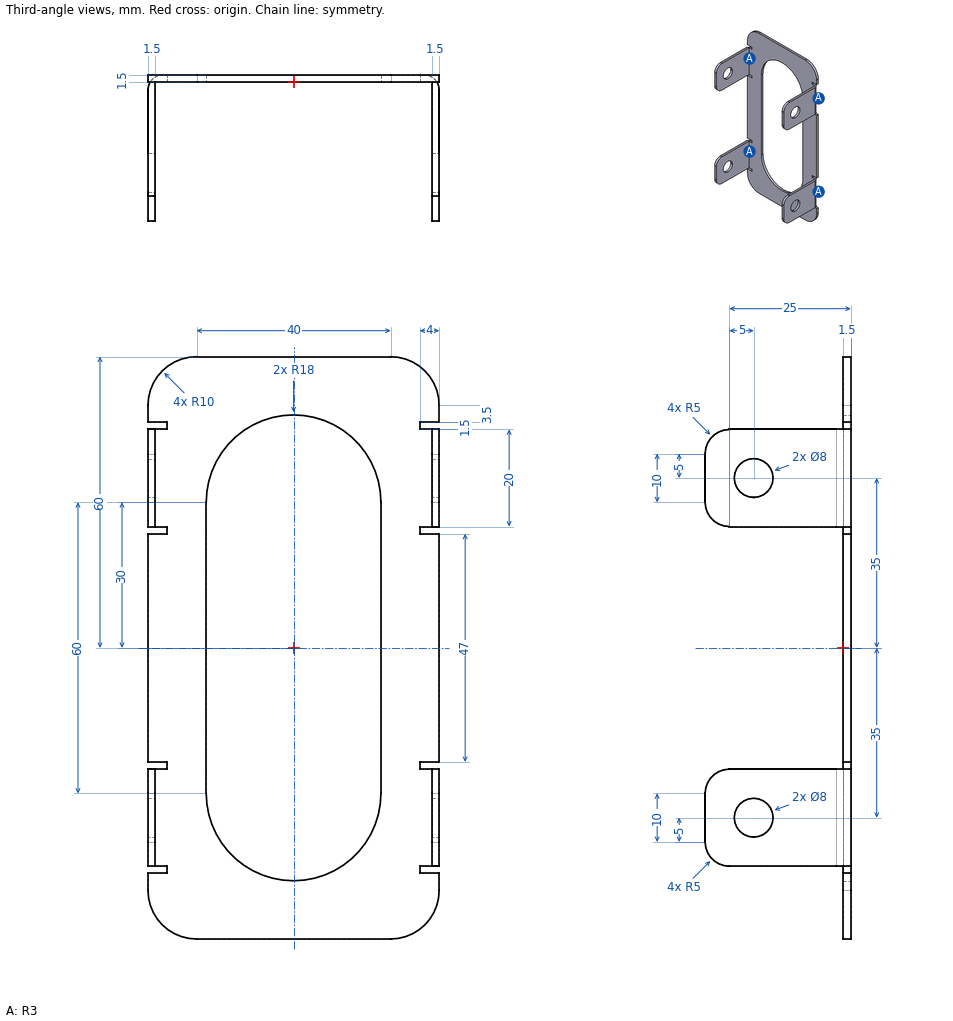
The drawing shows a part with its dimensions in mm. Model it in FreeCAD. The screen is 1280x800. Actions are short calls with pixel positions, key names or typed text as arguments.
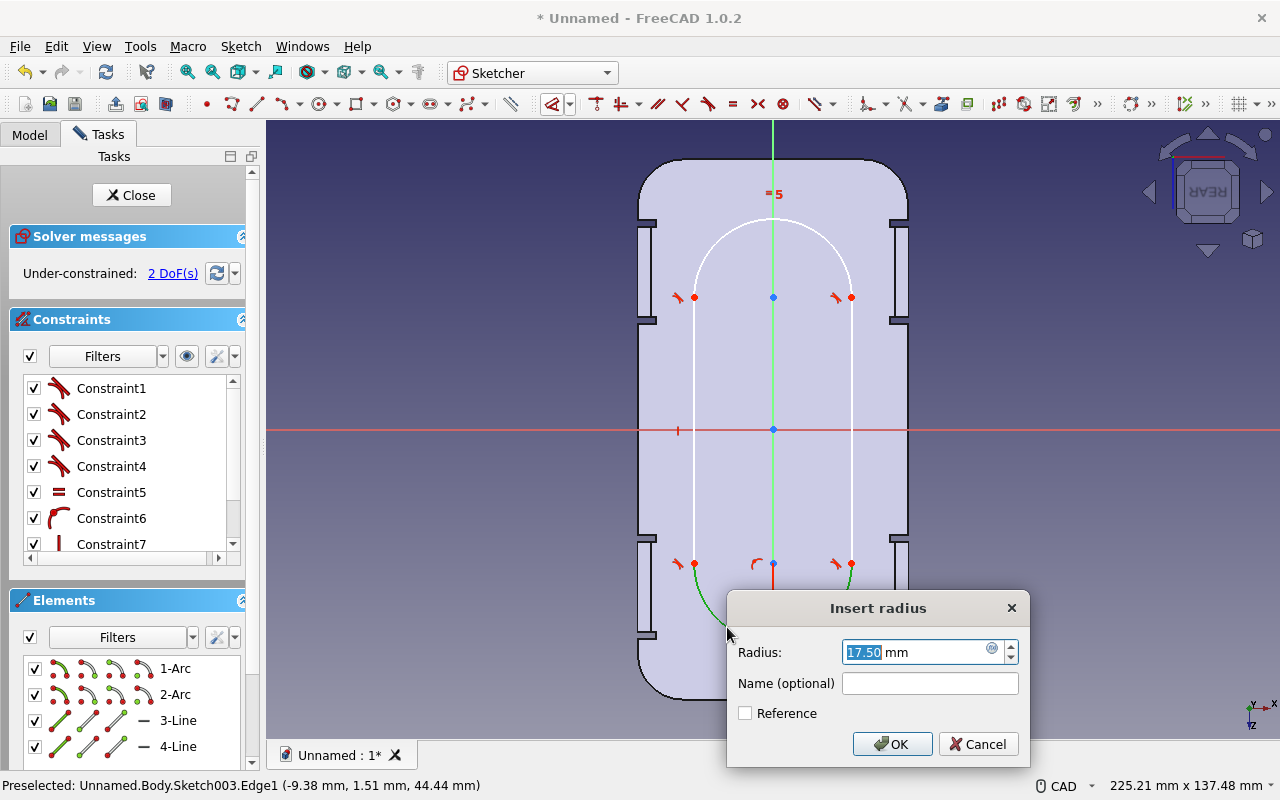
text(18)
key(Return)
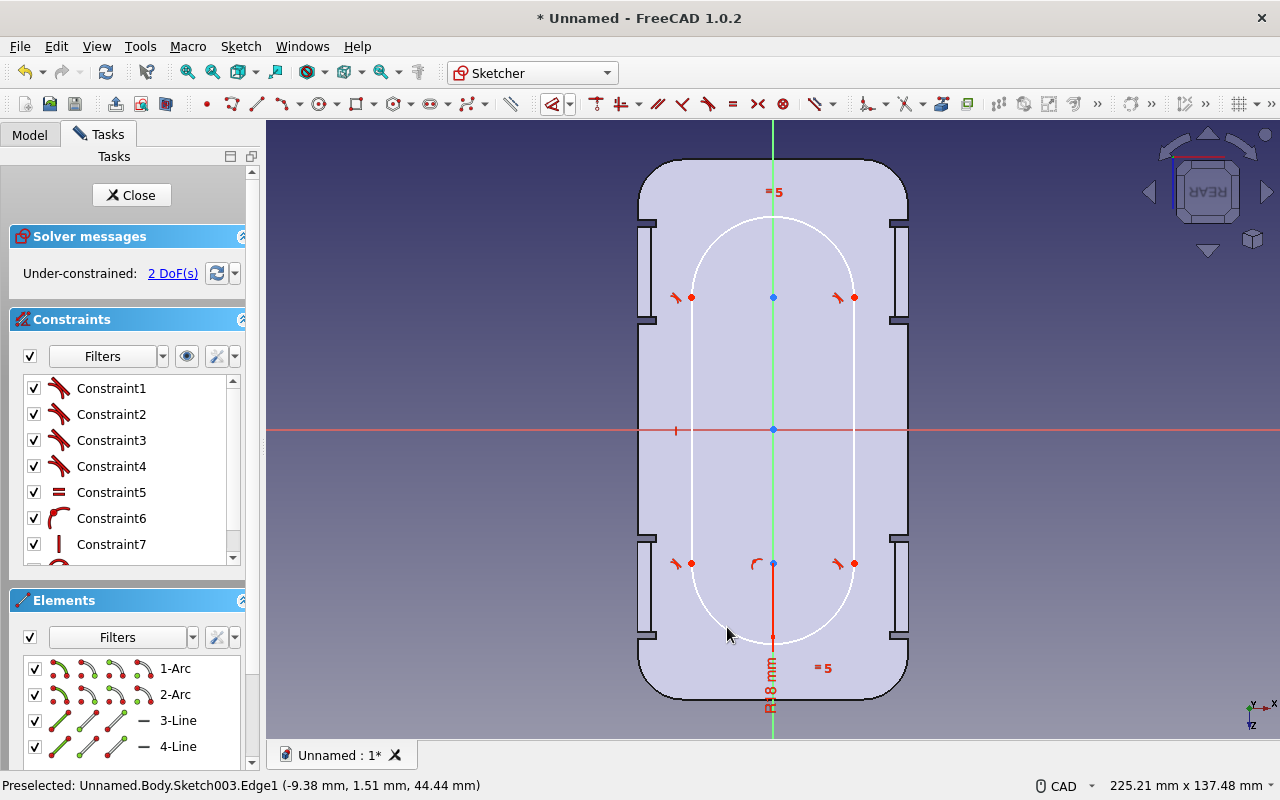
click(692, 484)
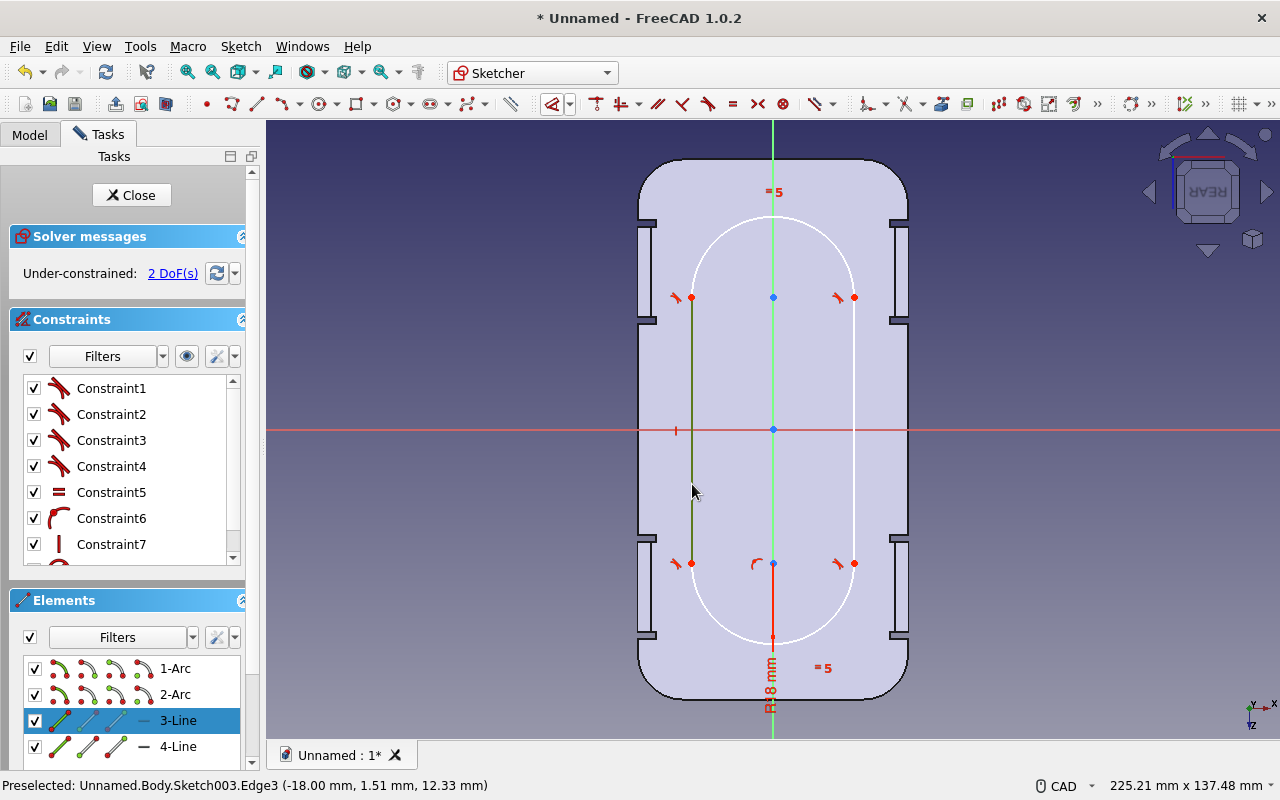
key(i)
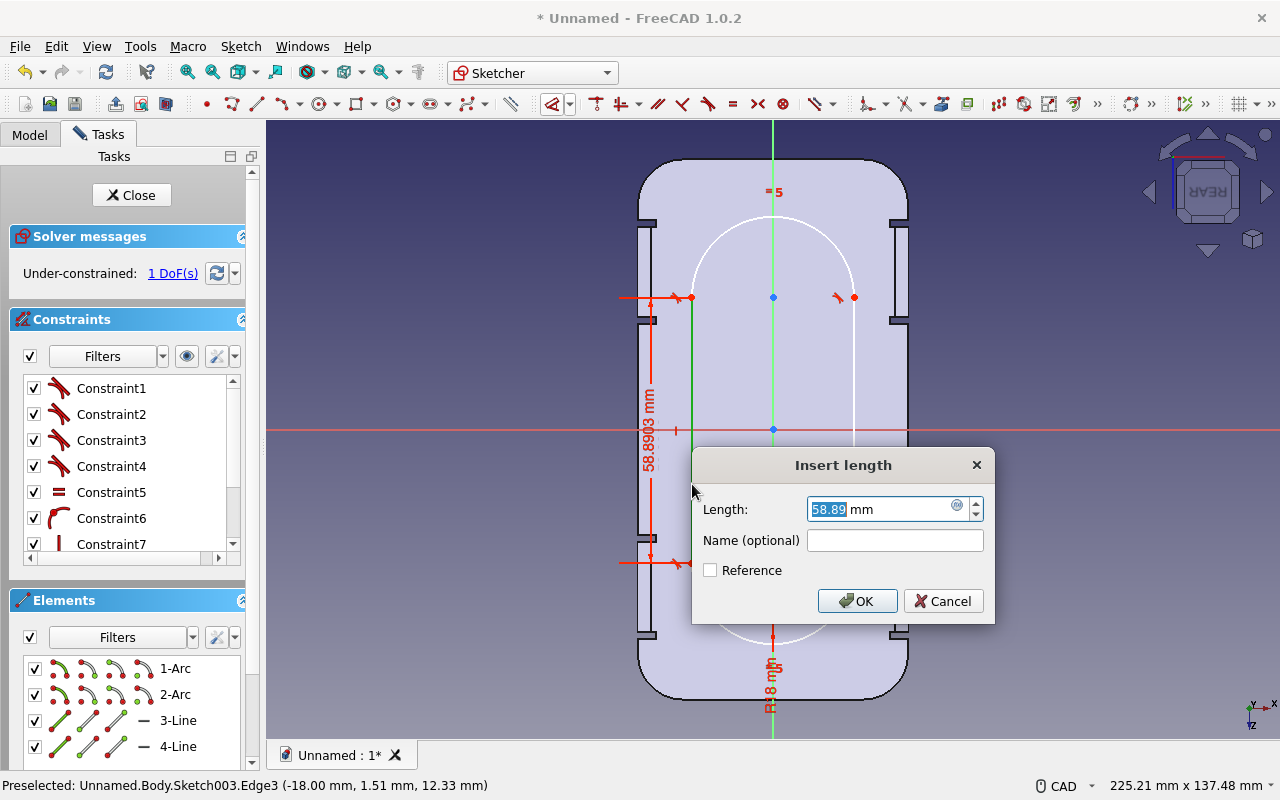
text(60)
key(Return)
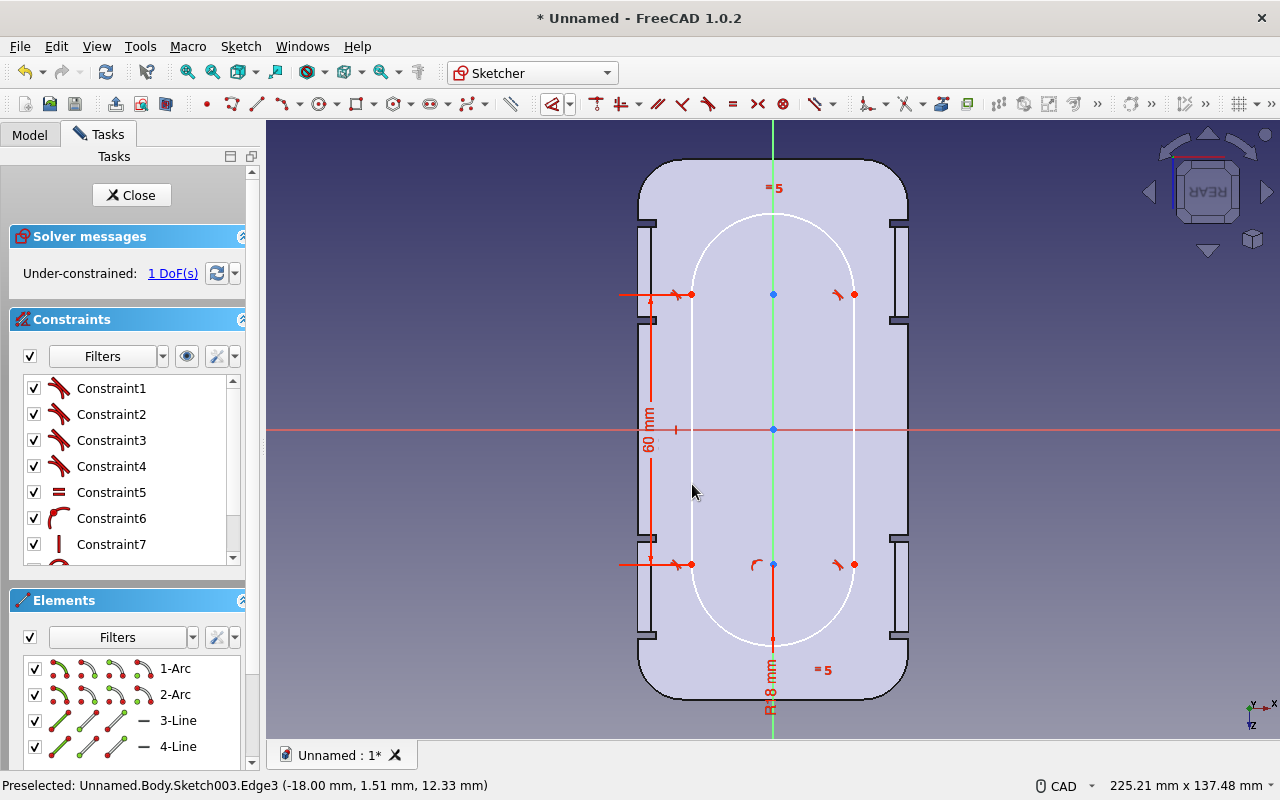
click(692, 565)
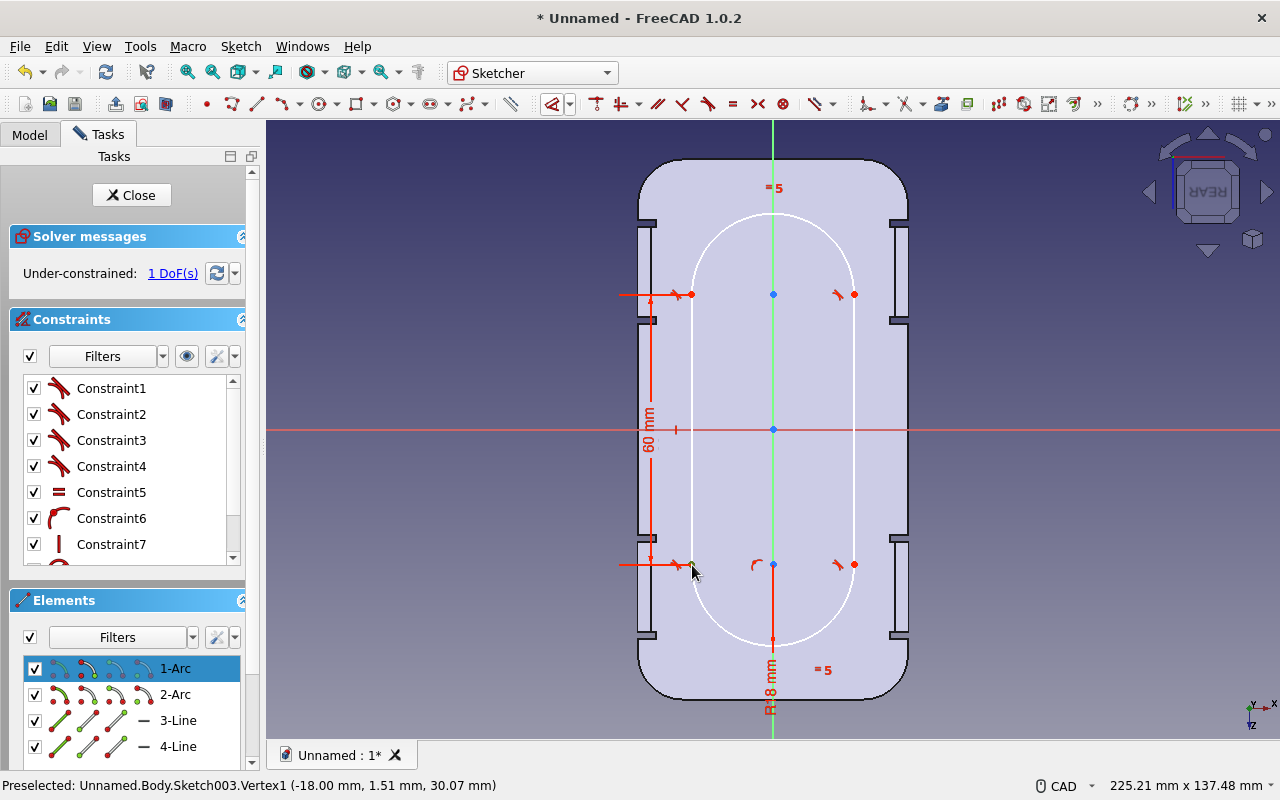
key(i)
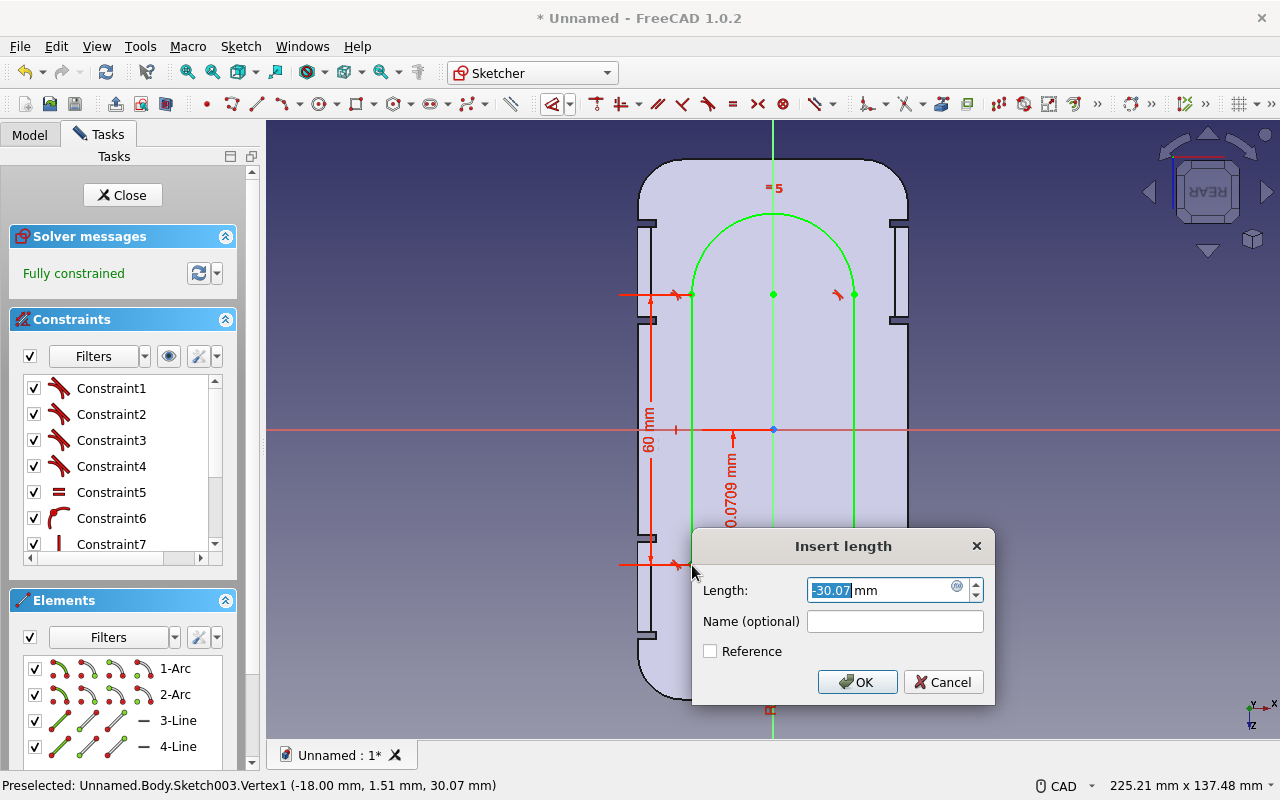
text(-30)
key(Return)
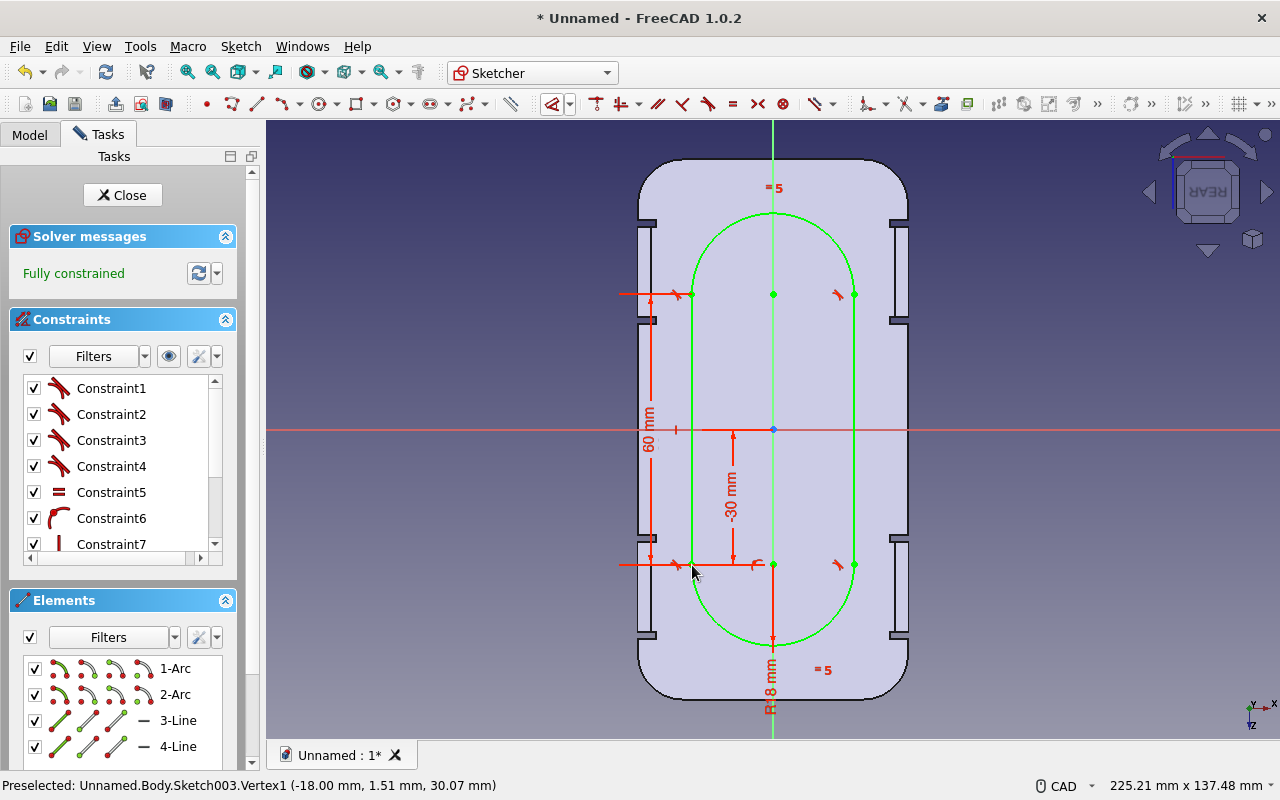
click(123, 195)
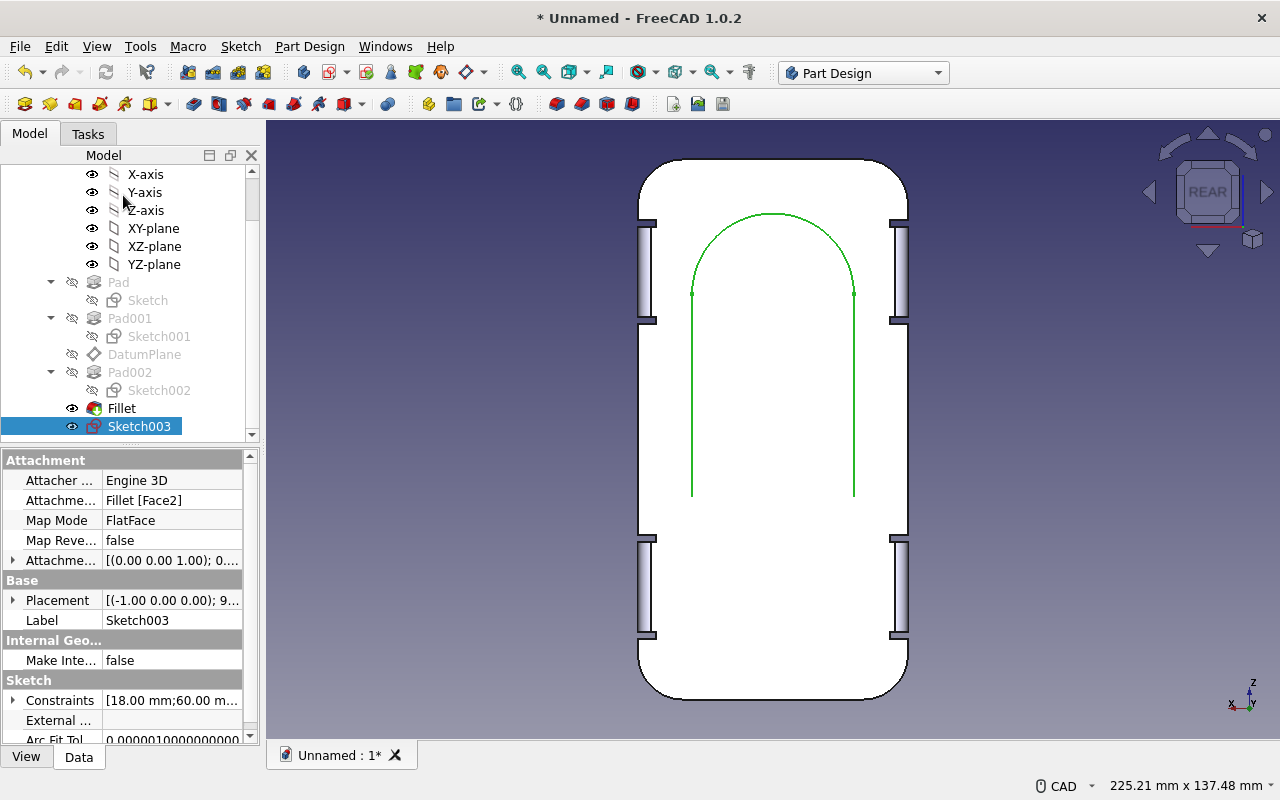
click(194, 104)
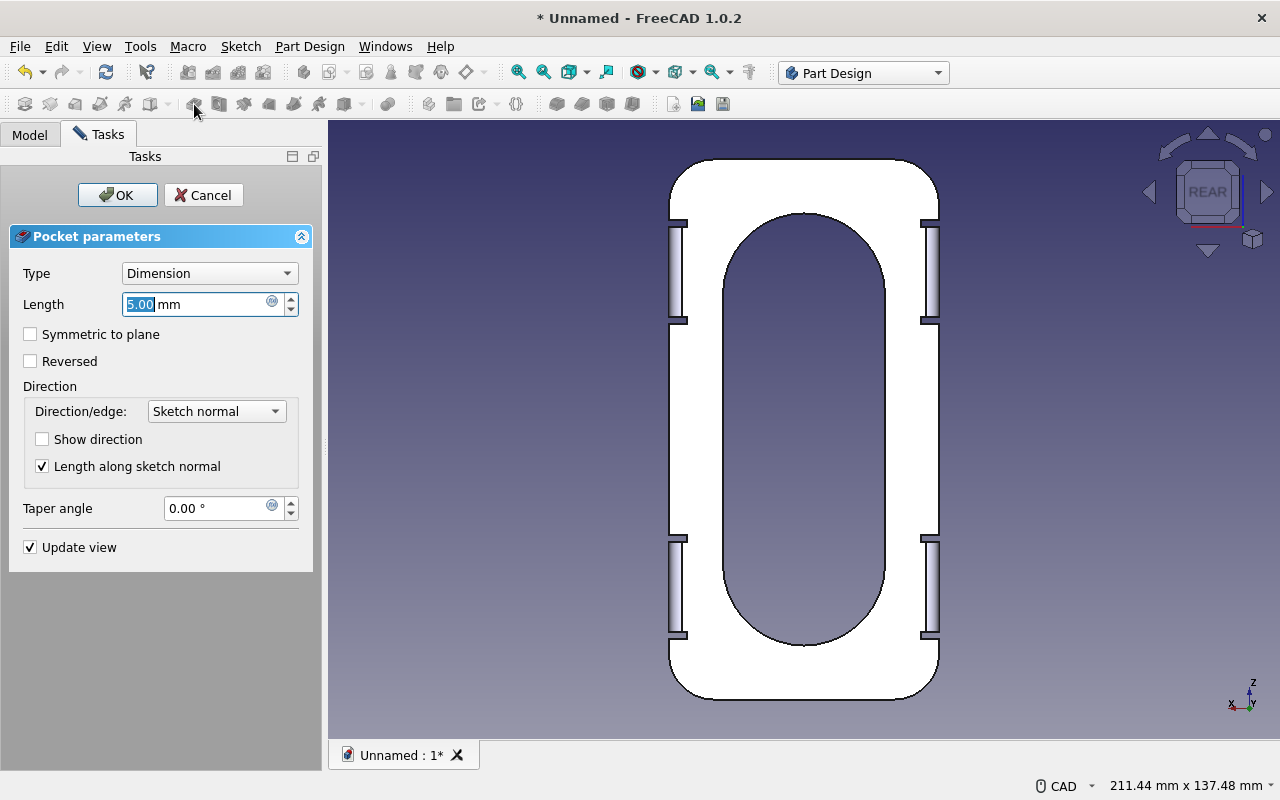
text(1.5)
key(Tab)